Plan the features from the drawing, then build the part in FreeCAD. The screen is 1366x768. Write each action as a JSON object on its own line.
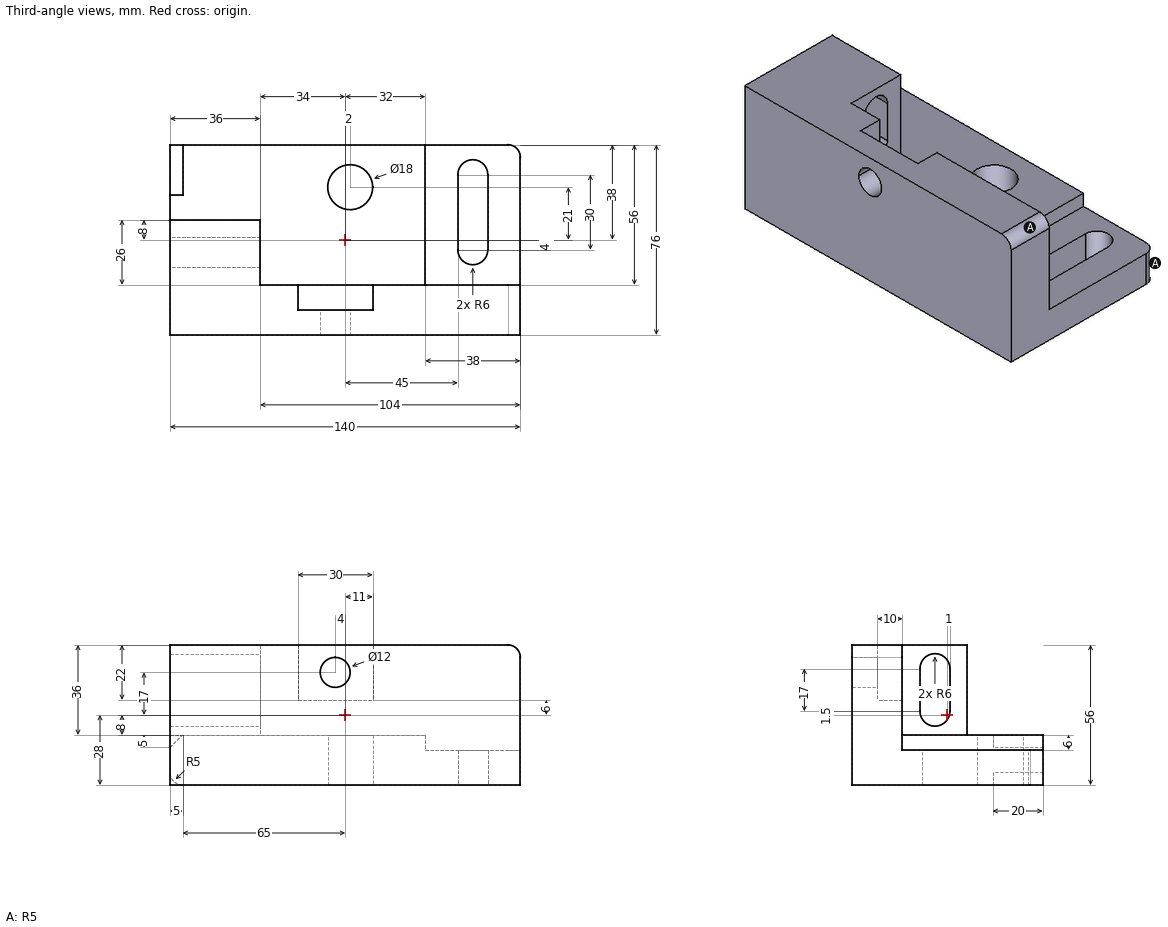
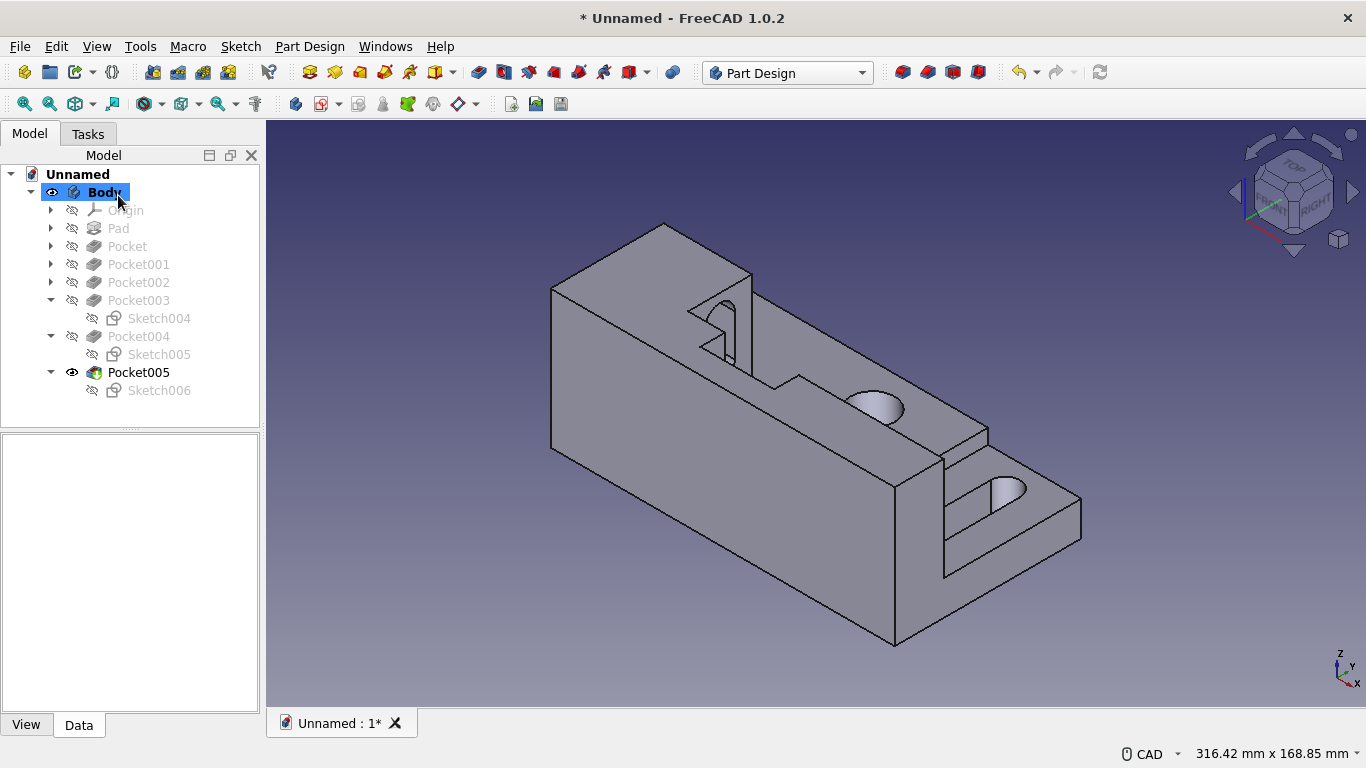
{"action": "key", "text": "4"}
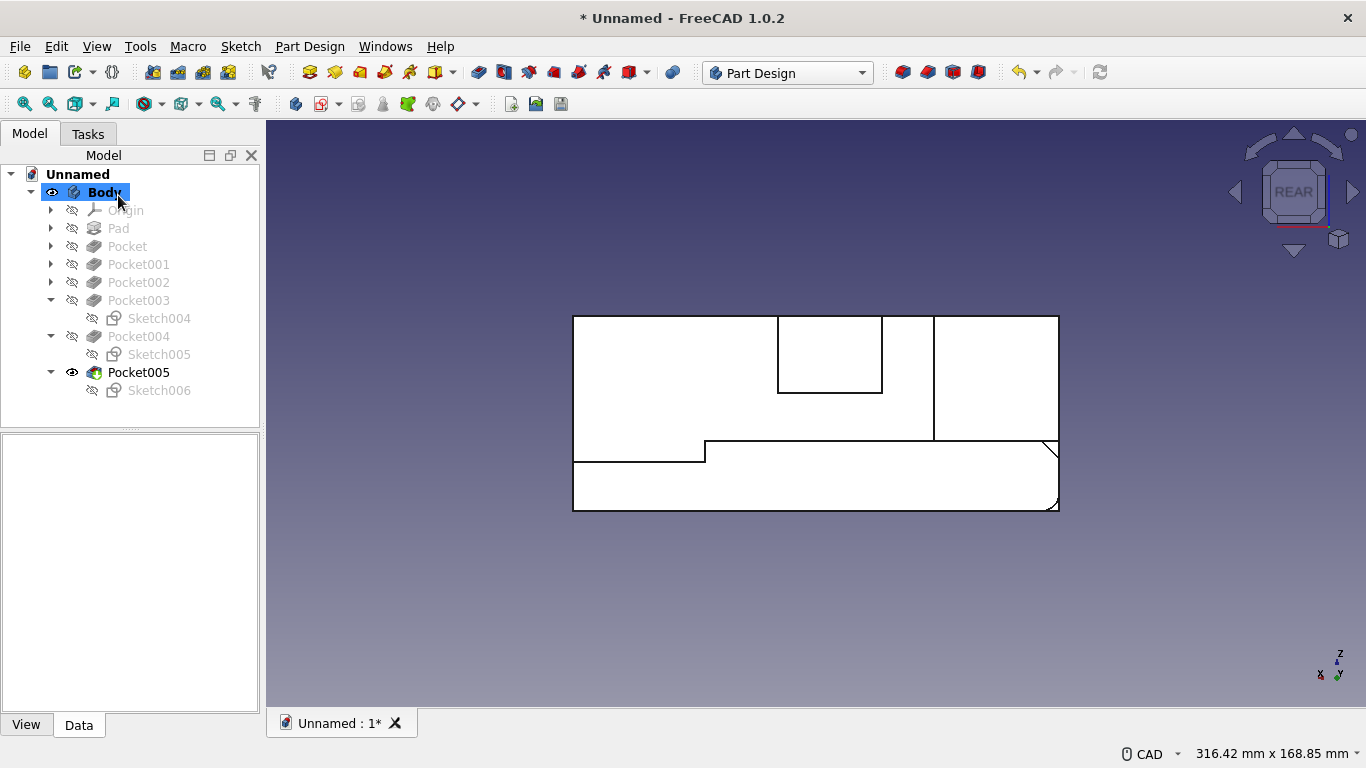
{"action": "left_click", "coordinate": [25, 104]}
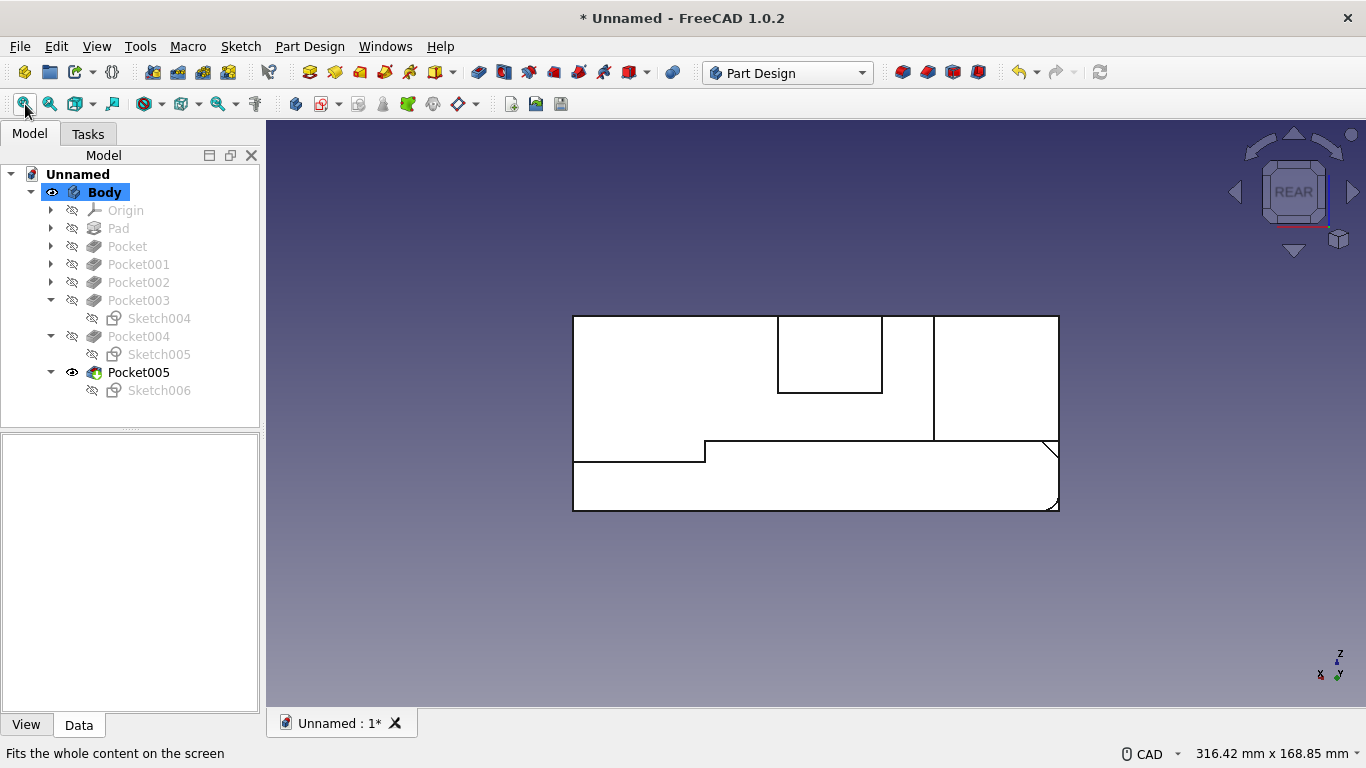
{"action": "left_click", "coordinate": [830, 353]}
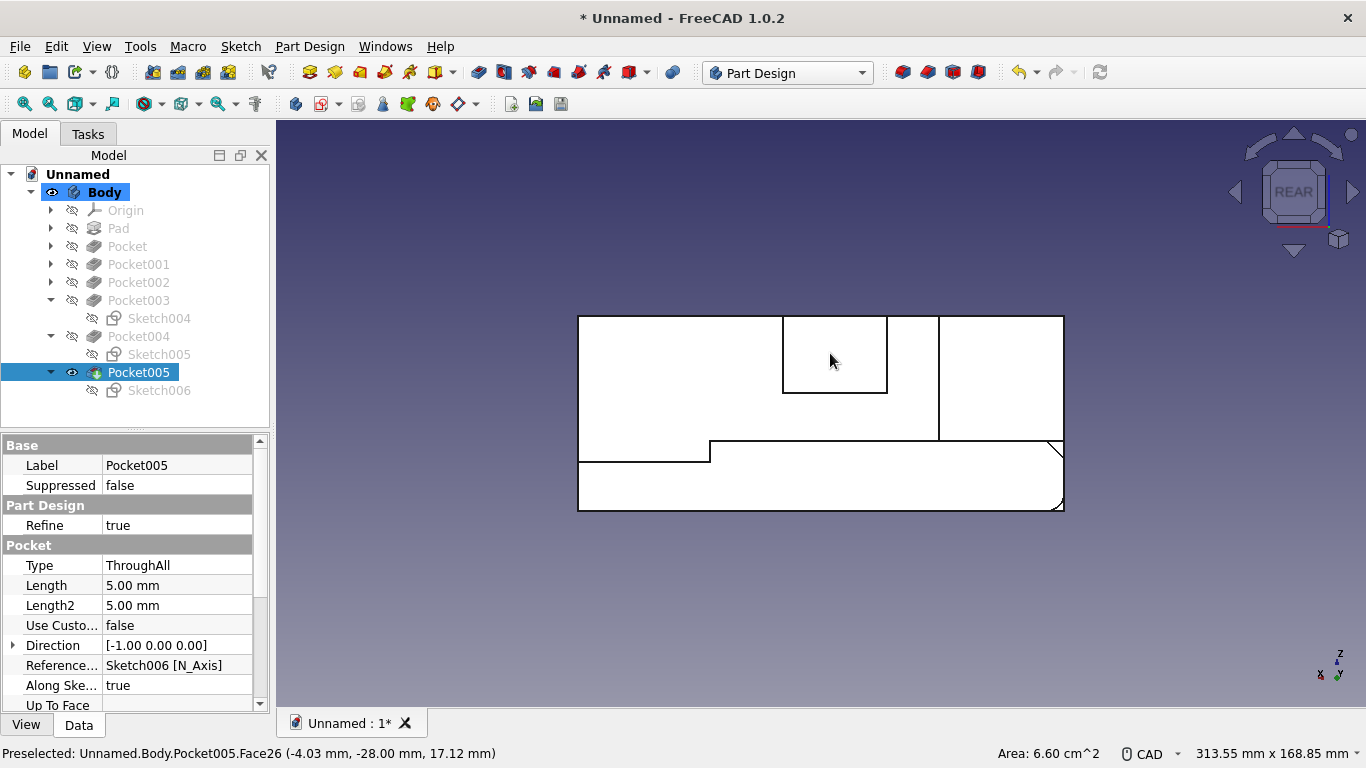
{"action": "left_click", "coordinate": [320, 104]}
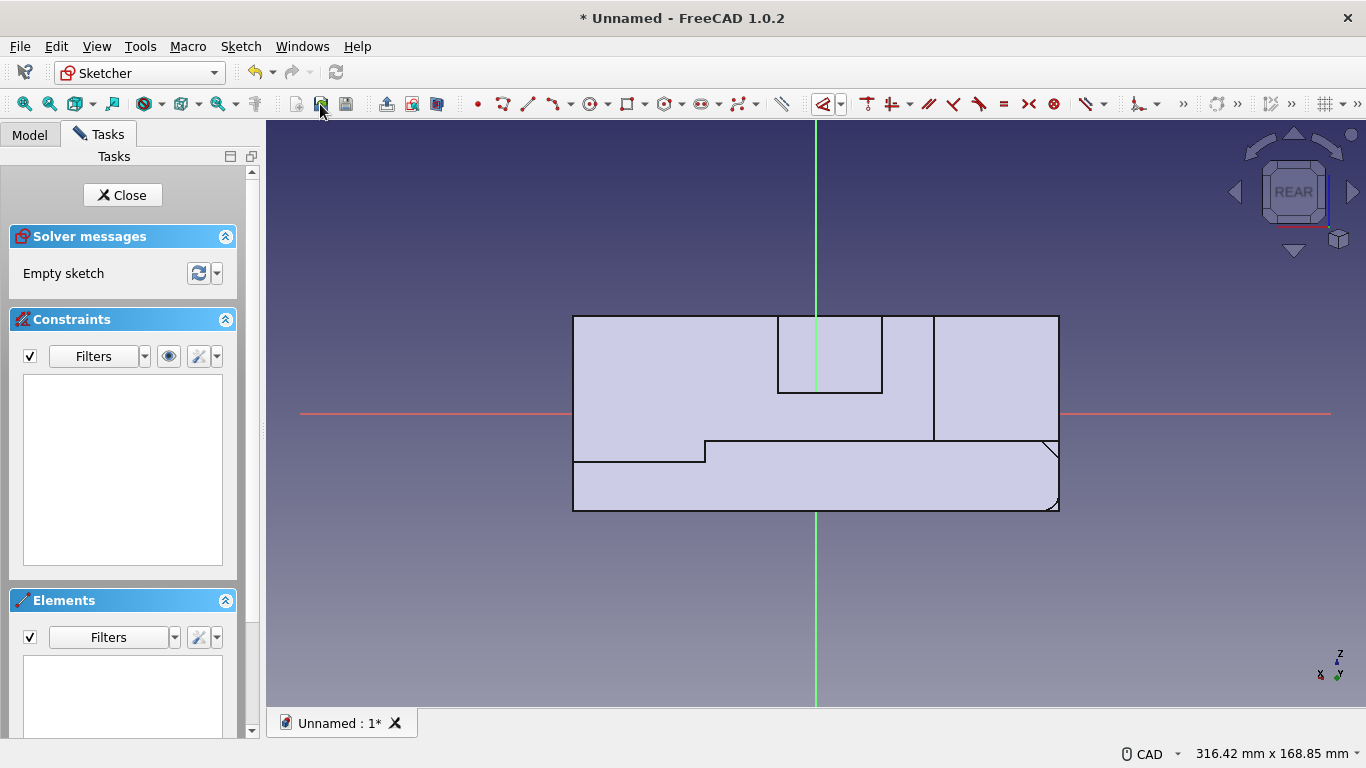
{"action": "scroll", "coordinate": [851, 363], "scroll_direction": "up", "scroll_amount": 8}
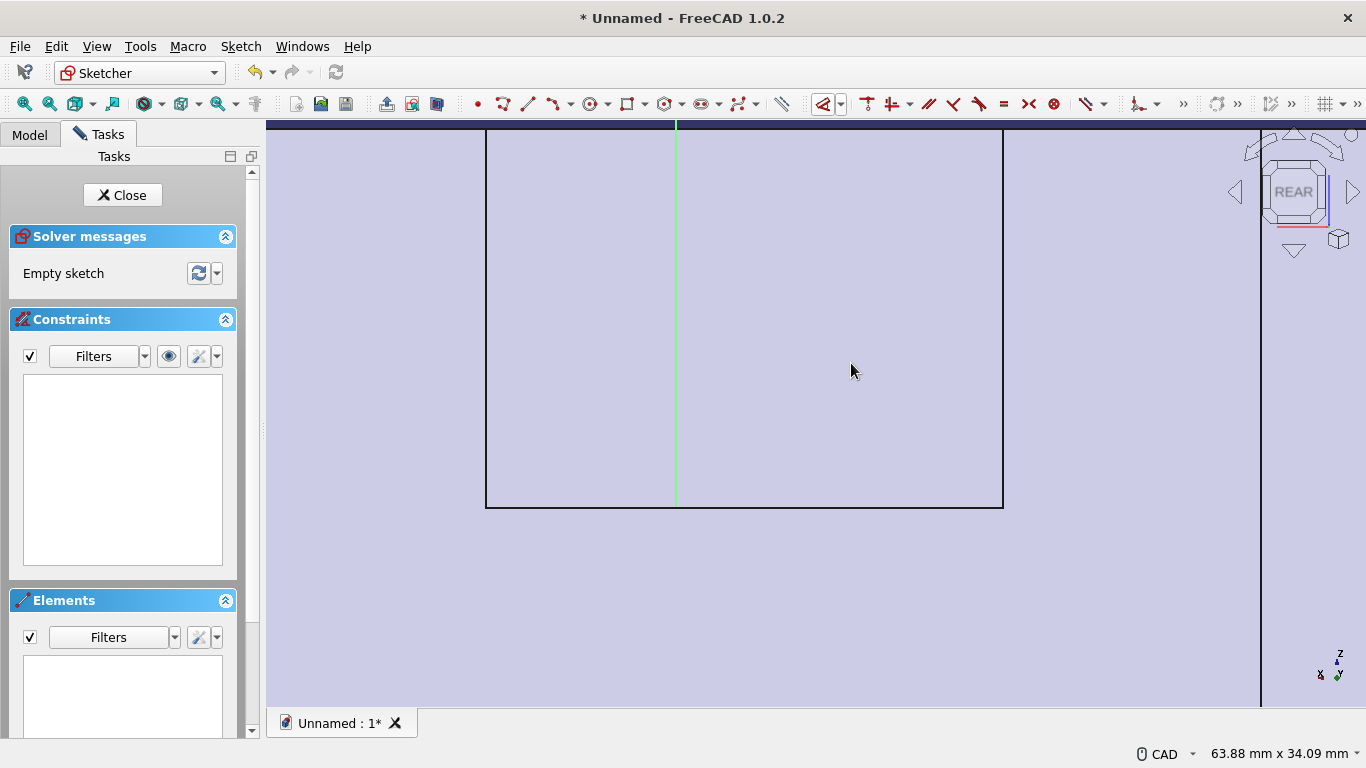
{"action": "left_click", "coordinate": [590, 104]}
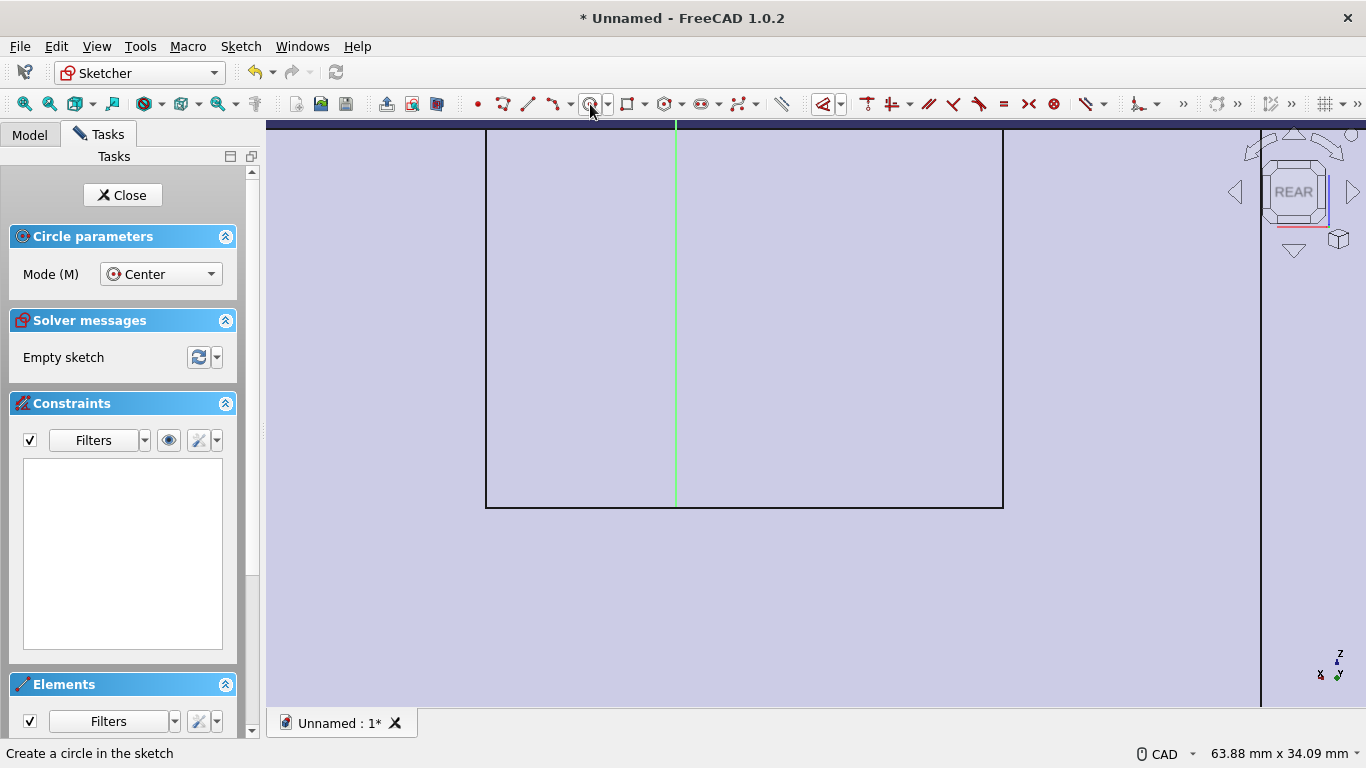
{"action": "left_click", "coordinate": [744, 319]}
{"action": "mouse_move", "coordinate": [817, 246]}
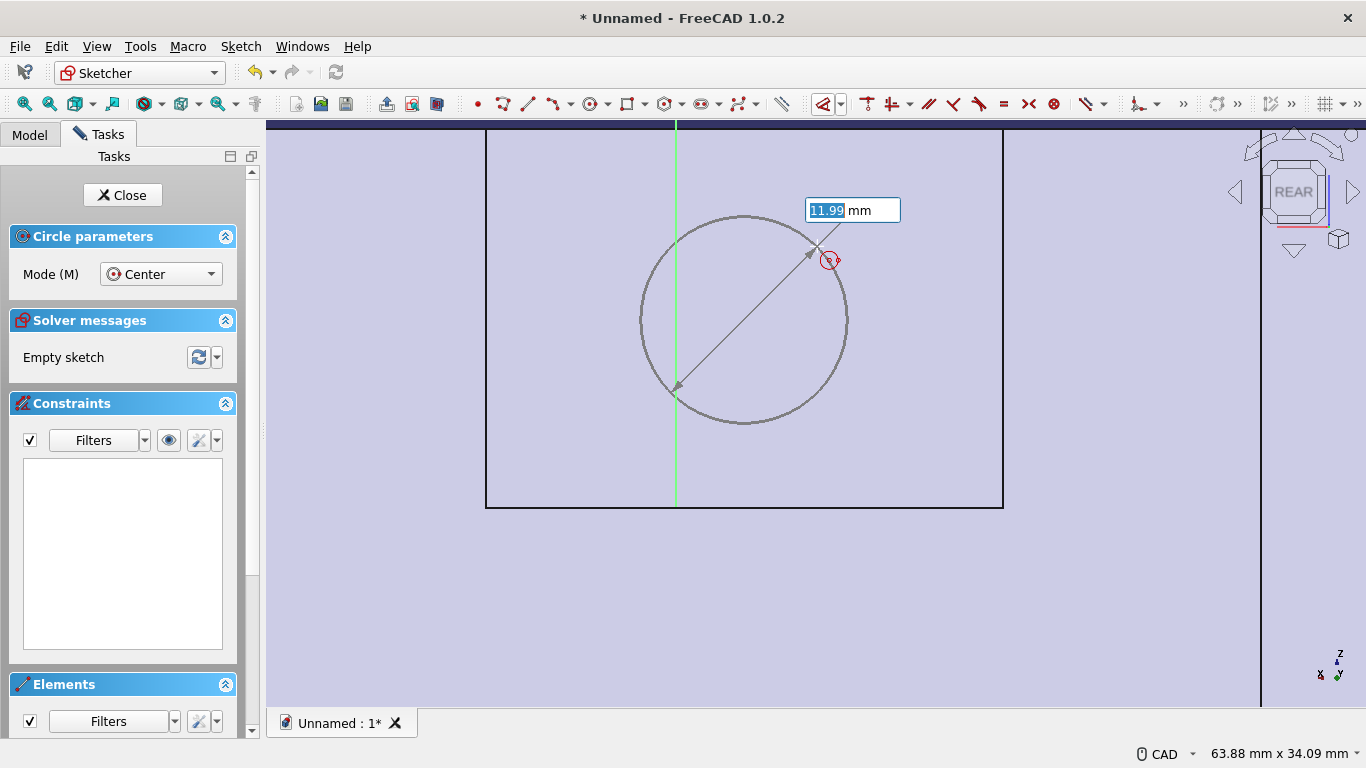
{"action": "type", "text": "12"}
{"action": "key", "text": "Return"}
{"action": "key", "text": "Escape"}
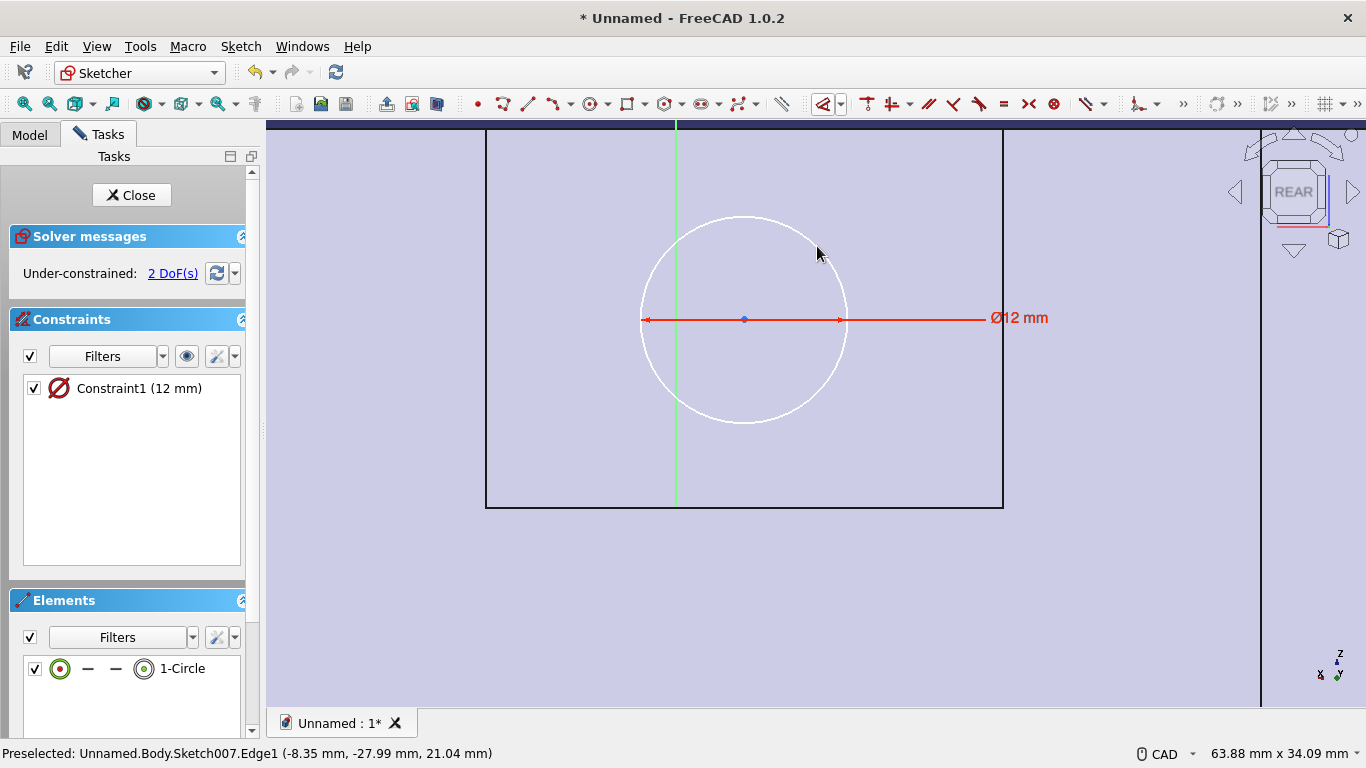
{"action": "left_click", "coordinate": [744, 320]}